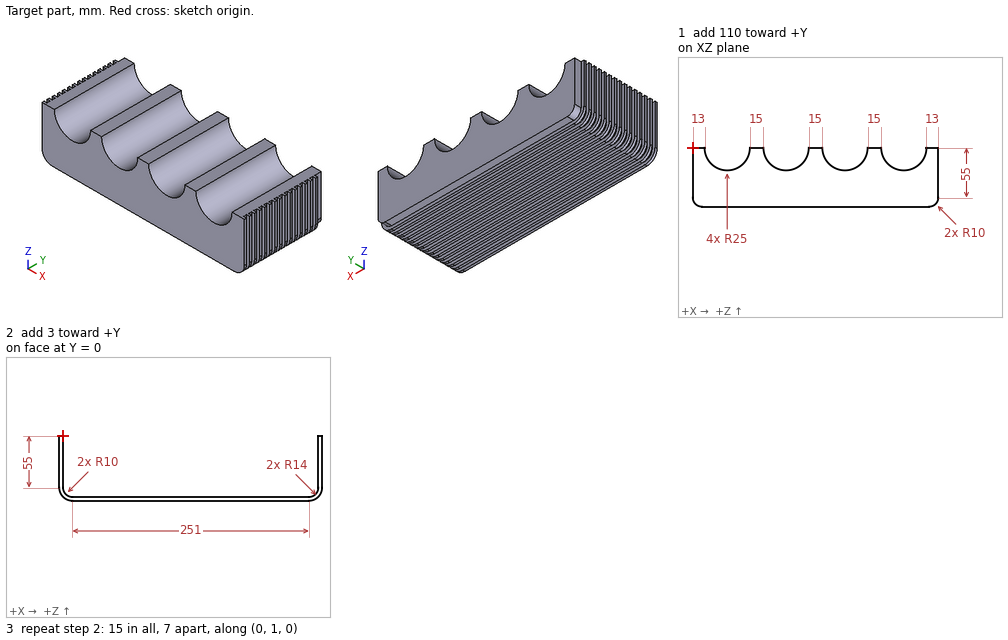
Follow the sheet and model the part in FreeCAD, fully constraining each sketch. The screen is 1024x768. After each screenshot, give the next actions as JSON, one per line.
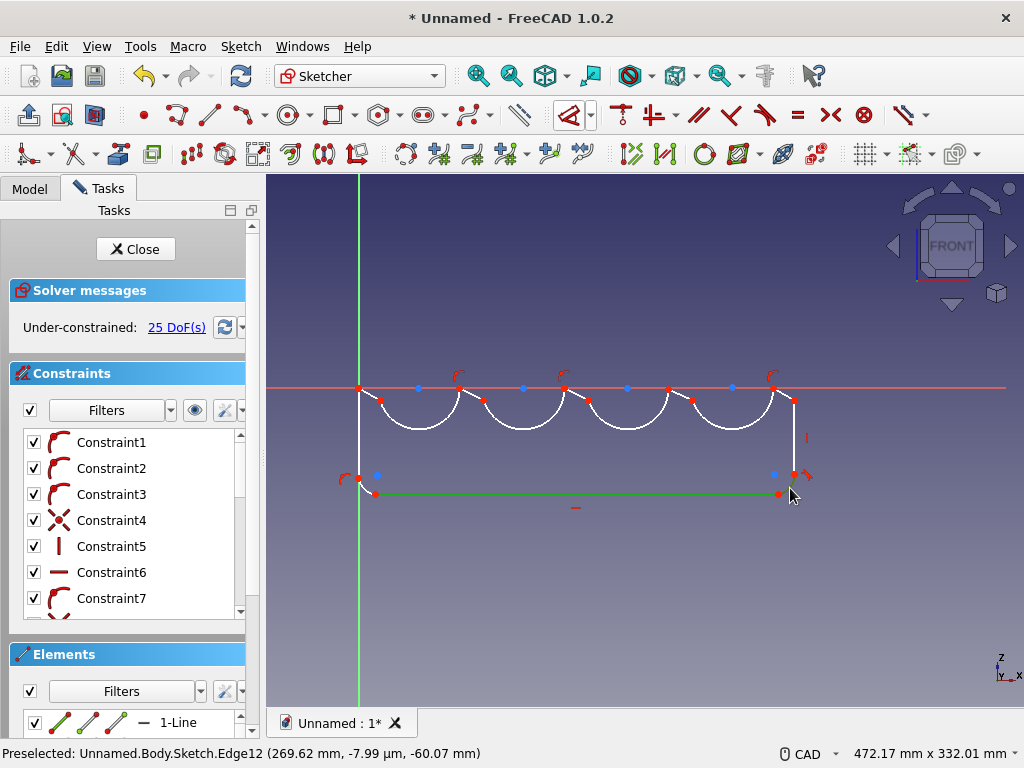
{"action": "left_click", "coordinate": [765, 116]}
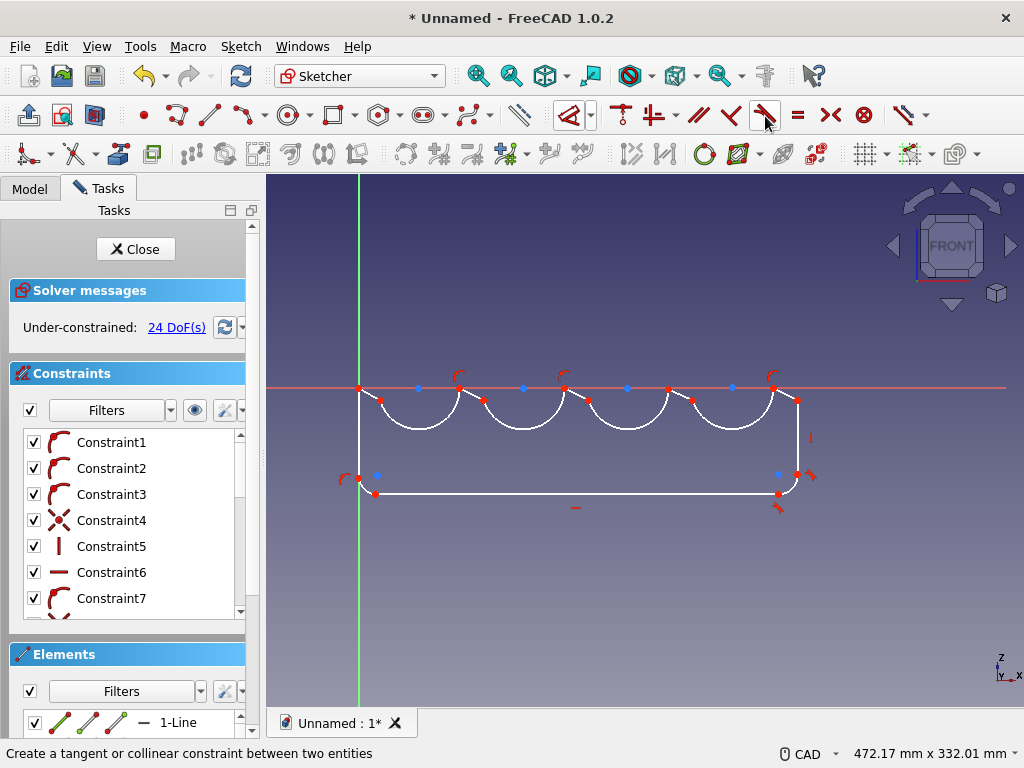
{"action": "left_click", "coordinate": [657, 494]}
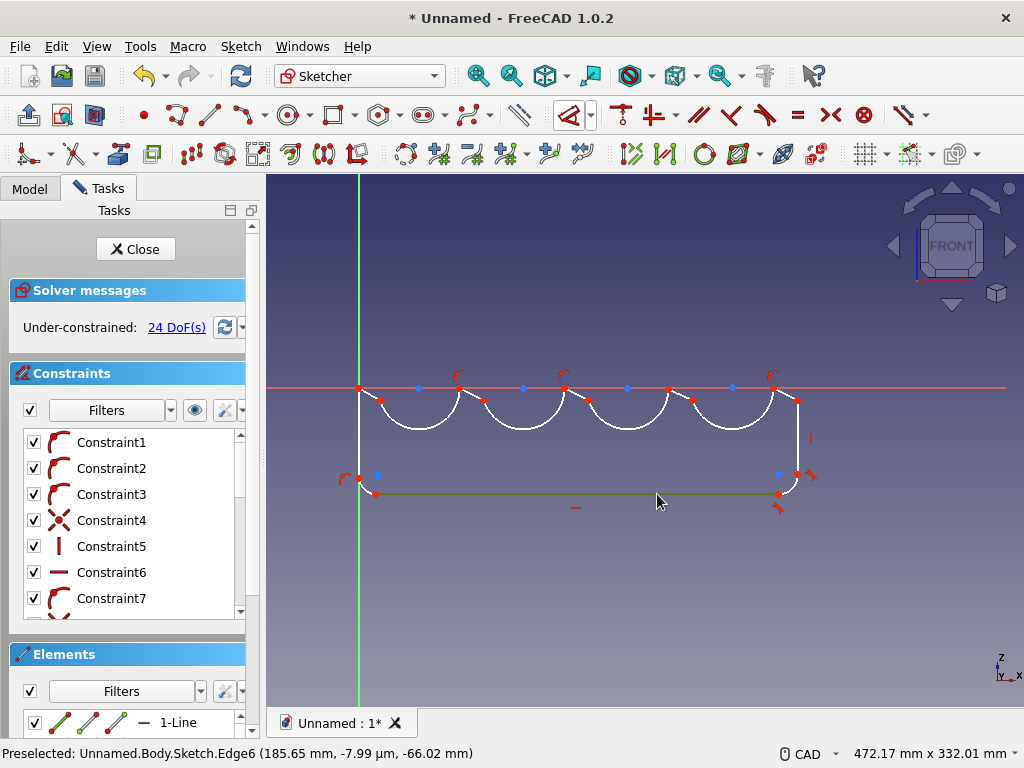
{"action": "scroll", "coordinate": [368, 492], "scroll_direction": "up", "scroll_amount": 4}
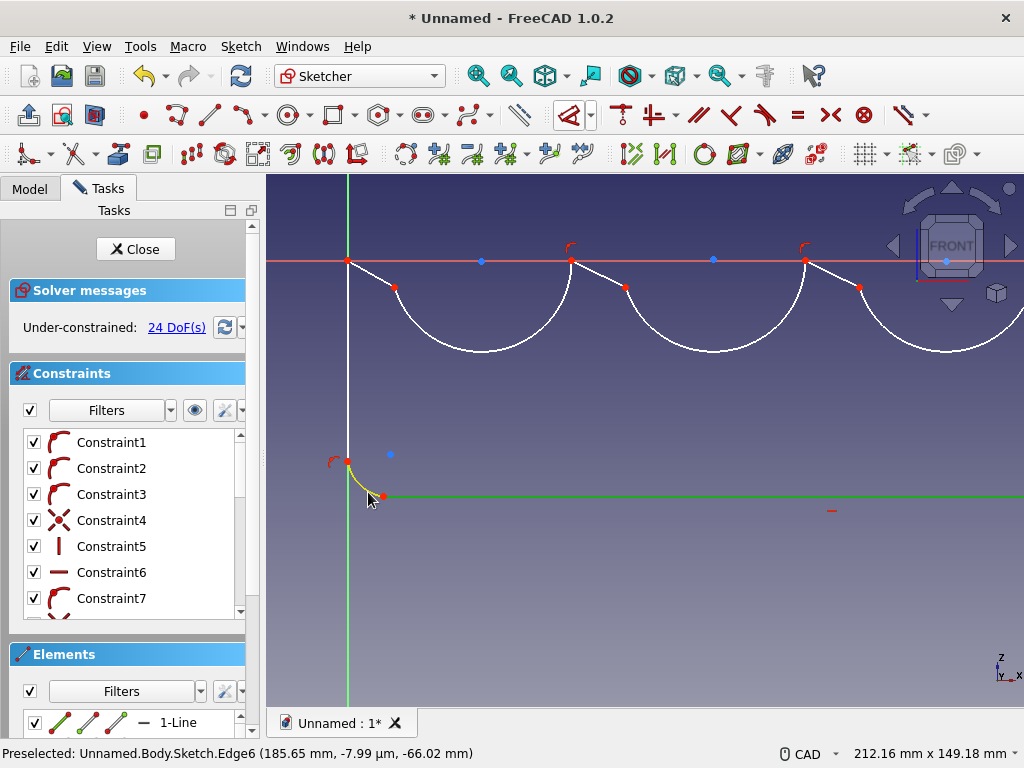
{"action": "left_click", "coordinate": [369, 491]}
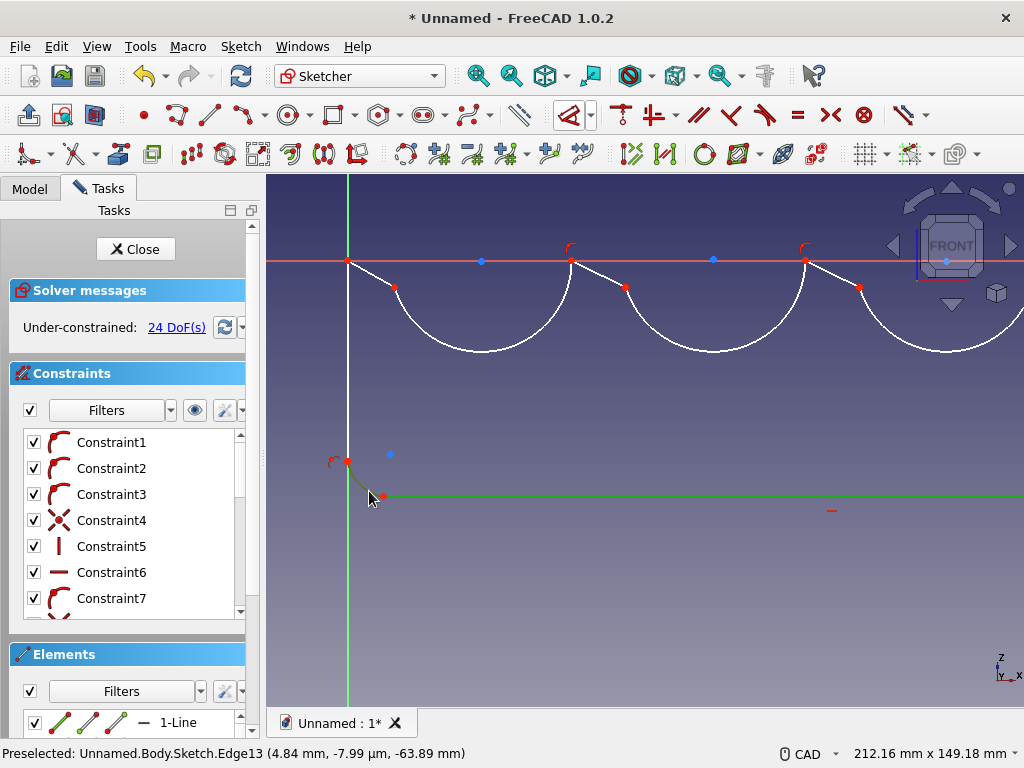
{"action": "left_click", "coordinate": [765, 116]}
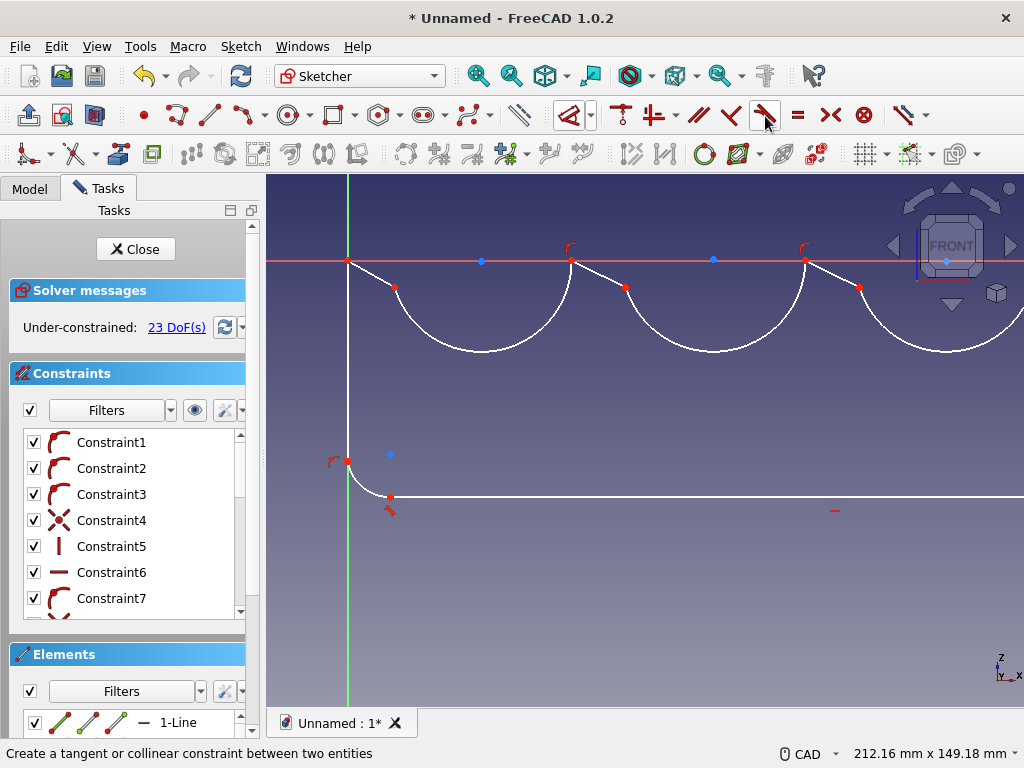
{"action": "left_click", "coordinate": [348, 401]}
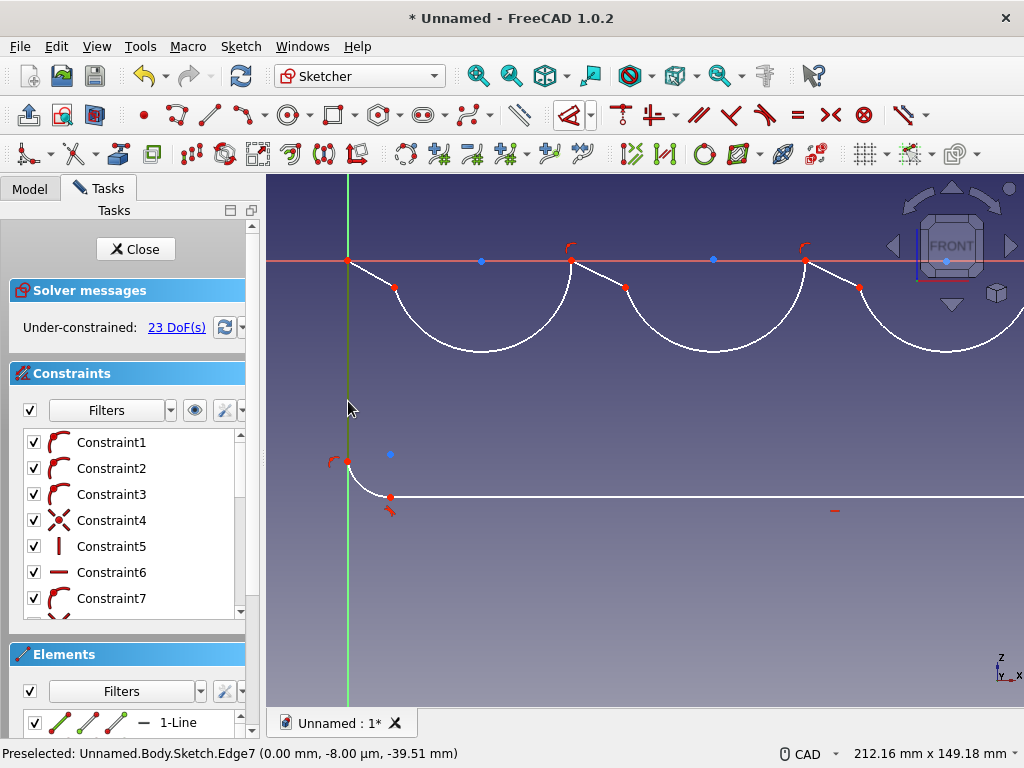
{"action": "left_click", "coordinate": [372, 493]}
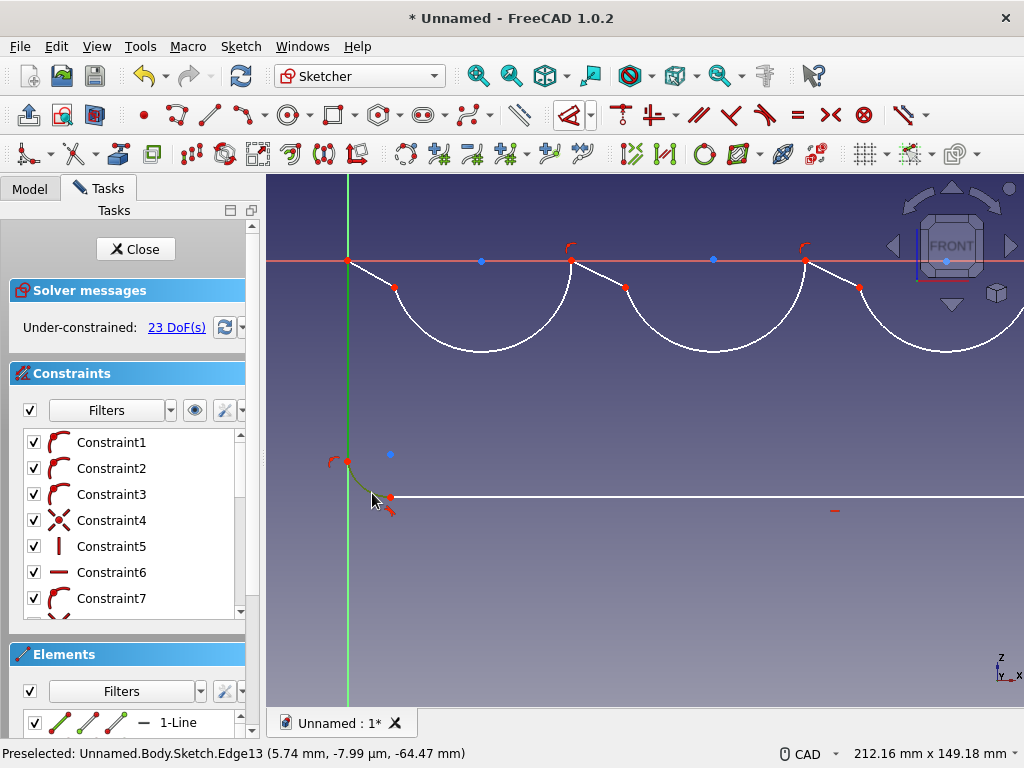
{"action": "left_click", "coordinate": [765, 116]}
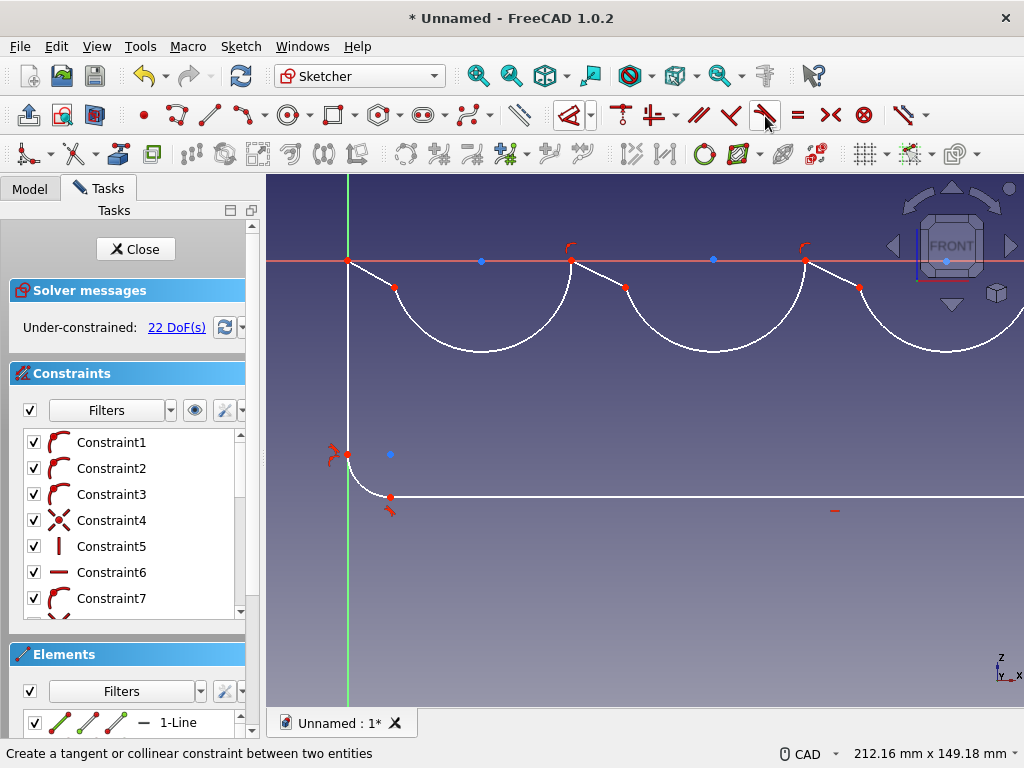
{"action": "left_click", "coordinate": [610, 279]}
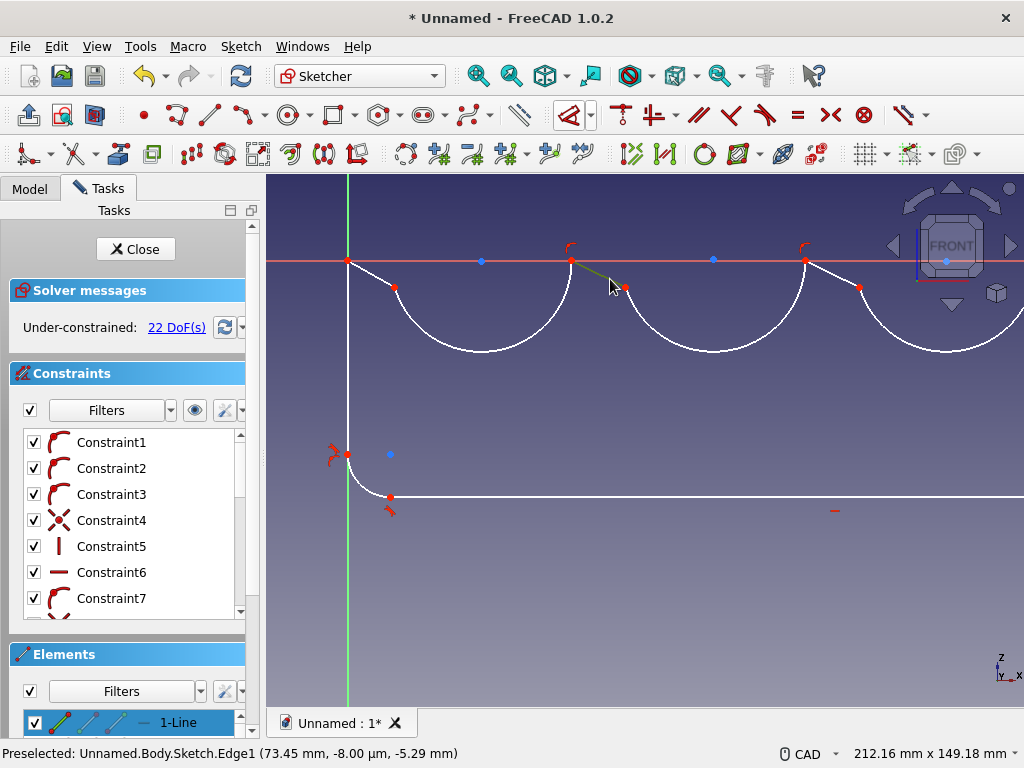
{"action": "left_click", "coordinate": [676, 116]}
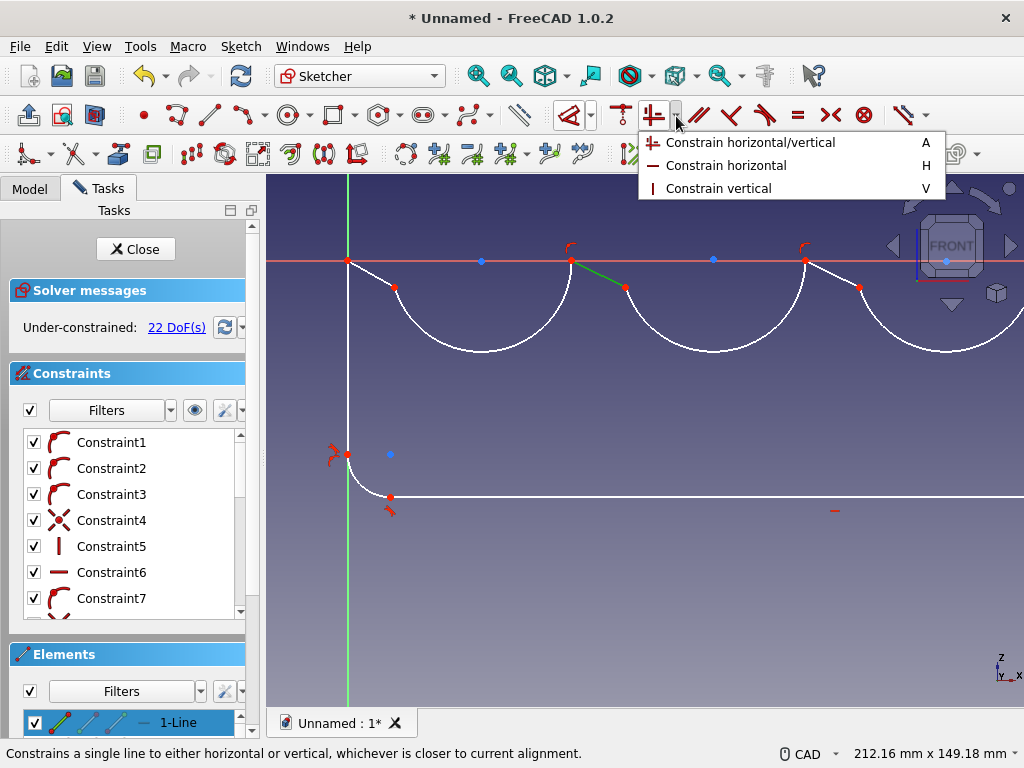
{"action": "left_click", "coordinate": [792, 166]}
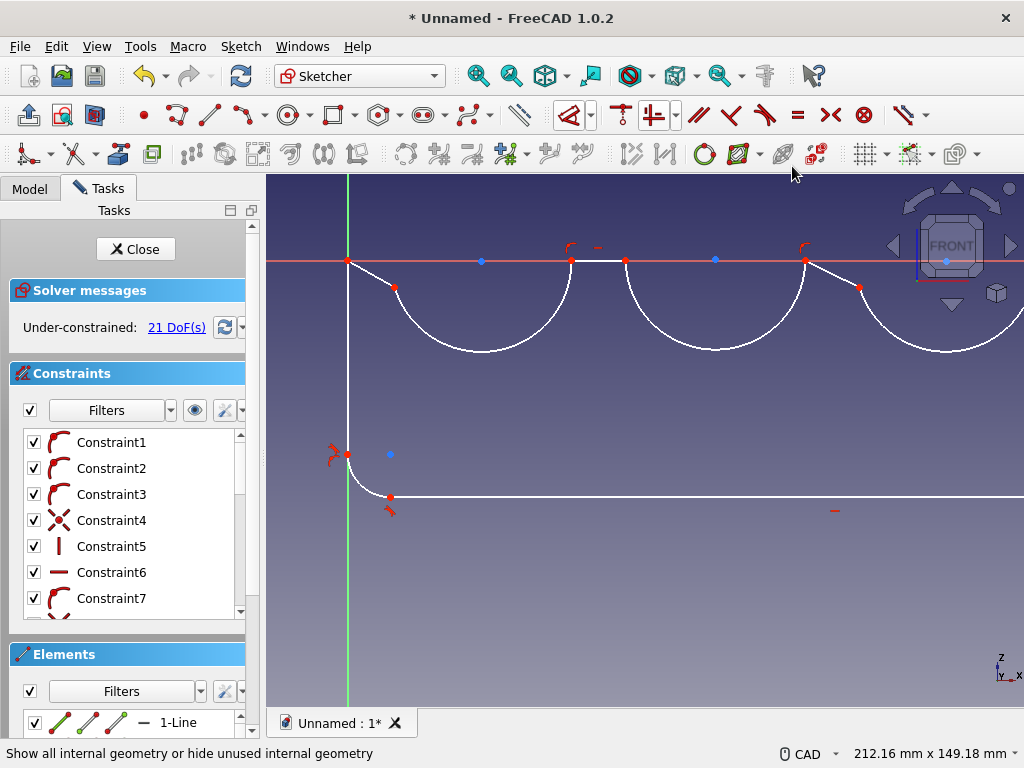
{"action": "left_click", "coordinate": [843, 279]}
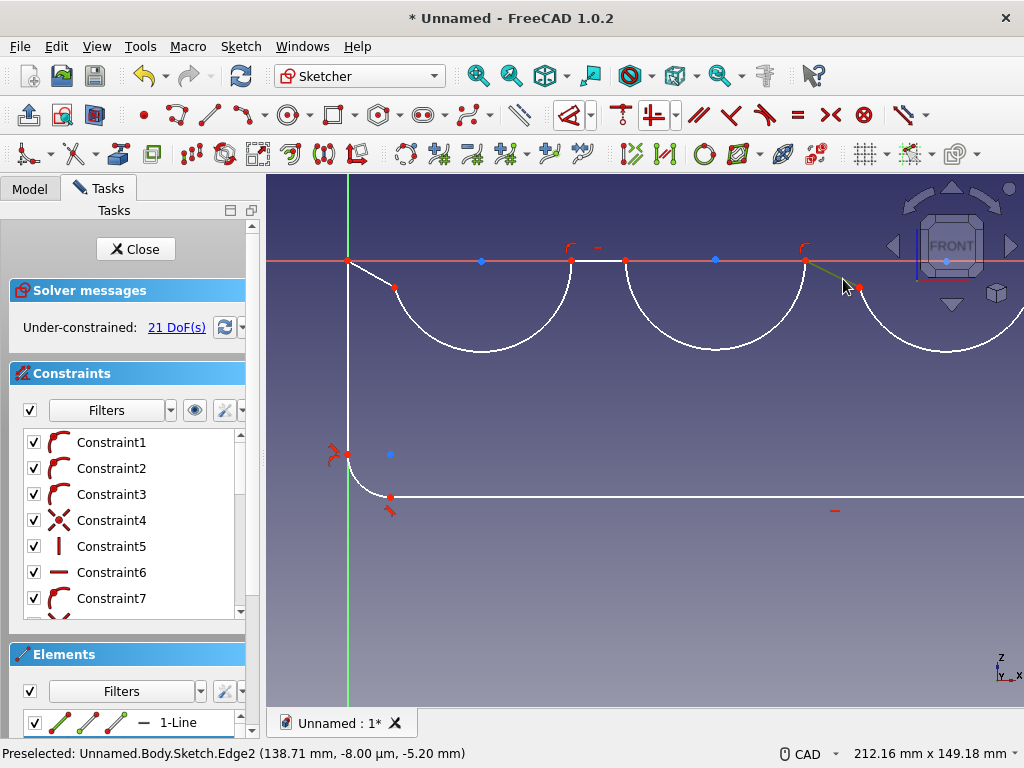
{"action": "key", "text": "h"}